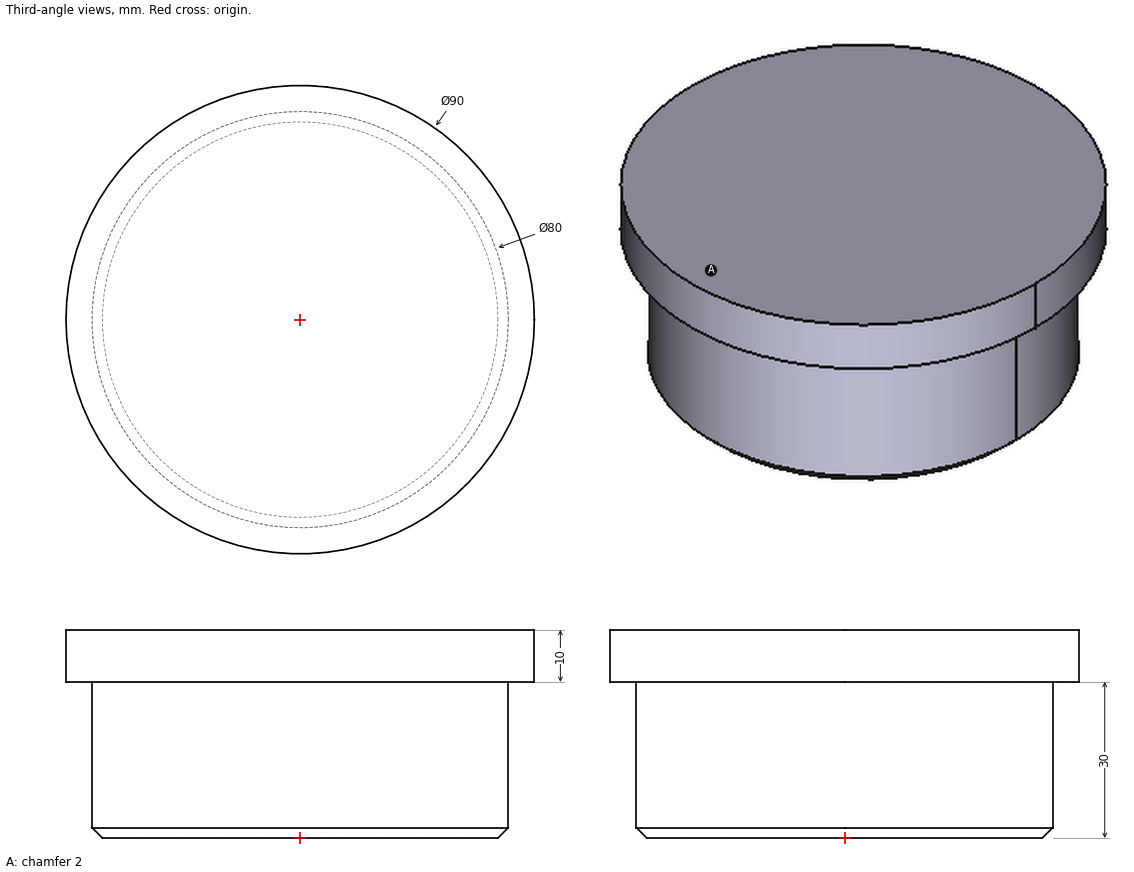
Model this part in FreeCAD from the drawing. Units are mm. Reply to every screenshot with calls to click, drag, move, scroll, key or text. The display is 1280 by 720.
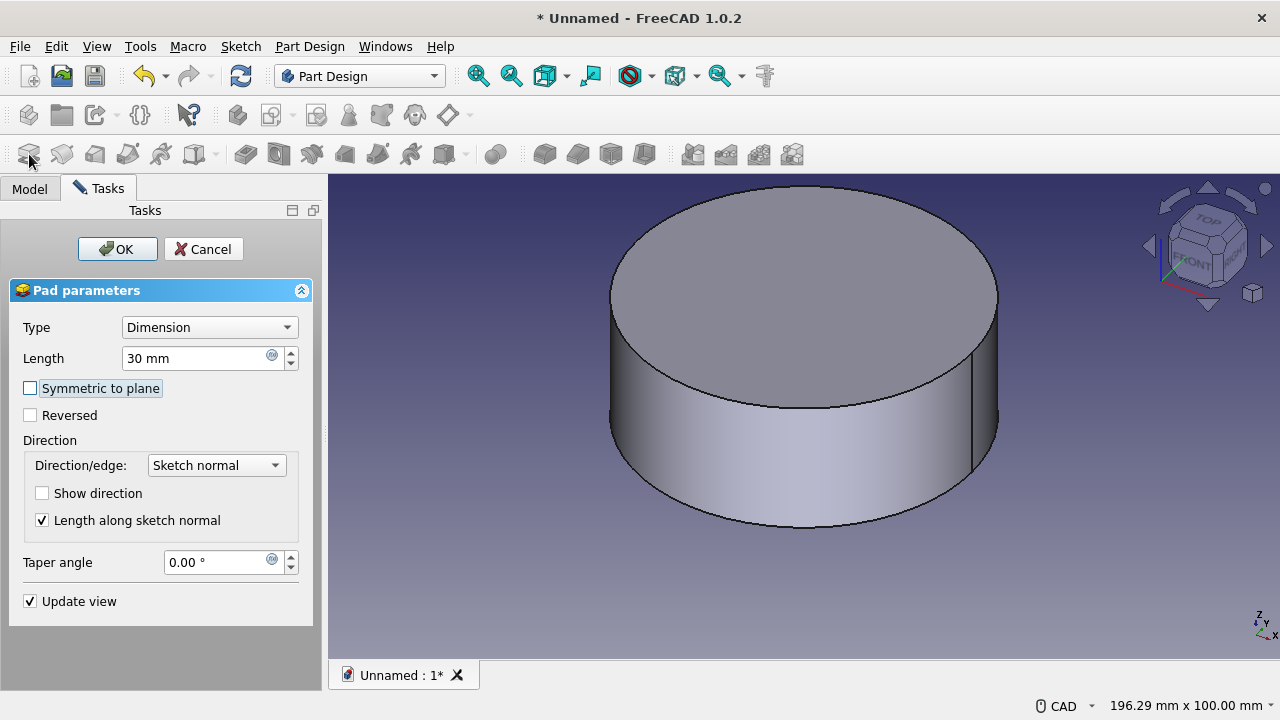
click(118, 249)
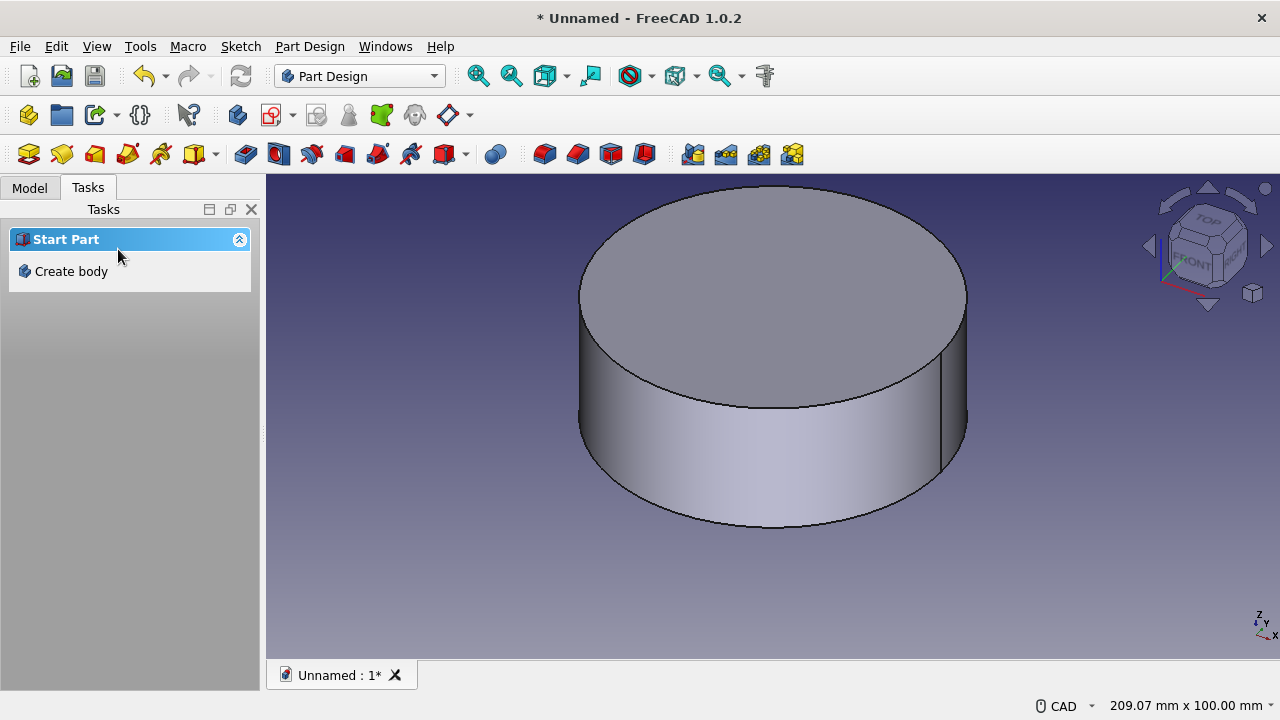
click(479, 76)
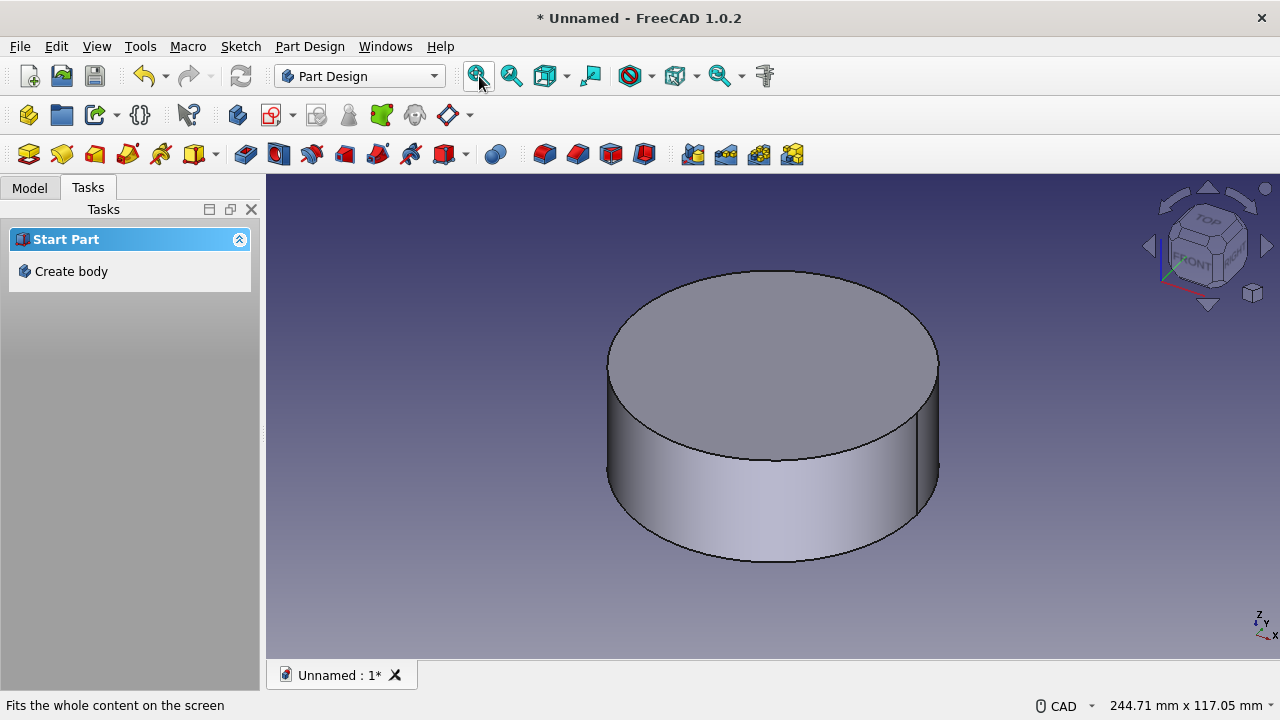
click(773, 365)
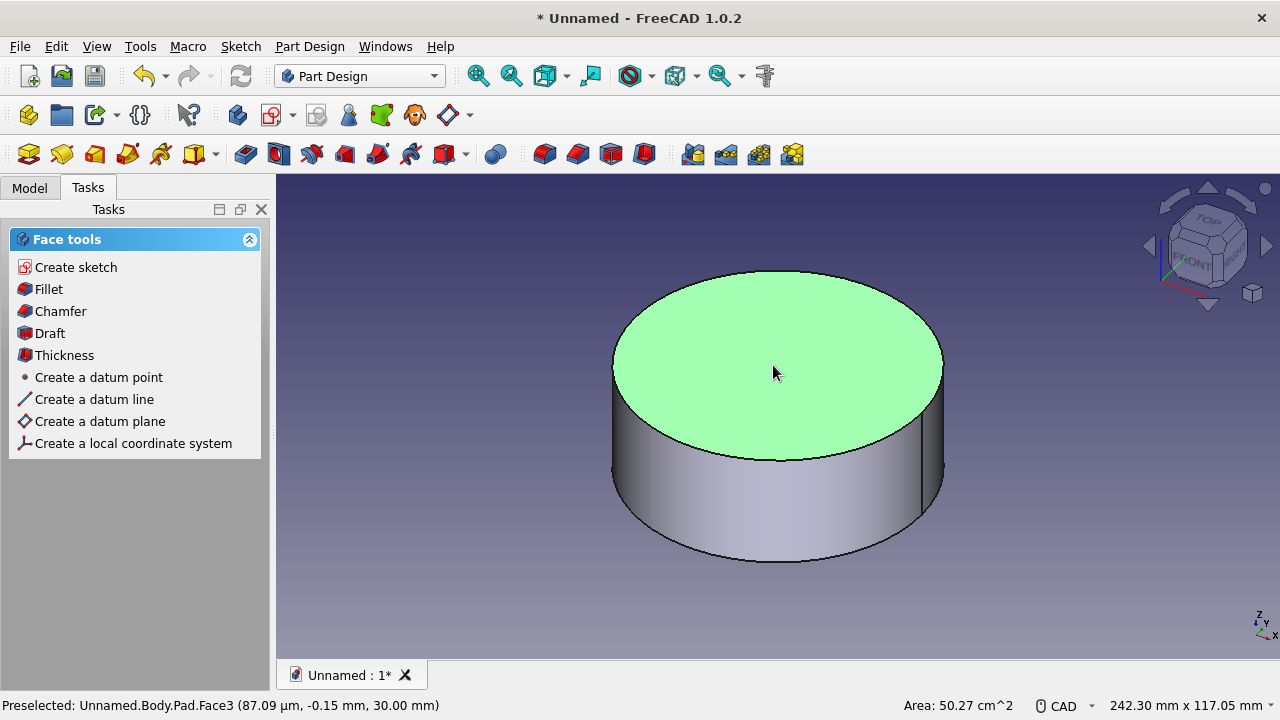
click(270, 116)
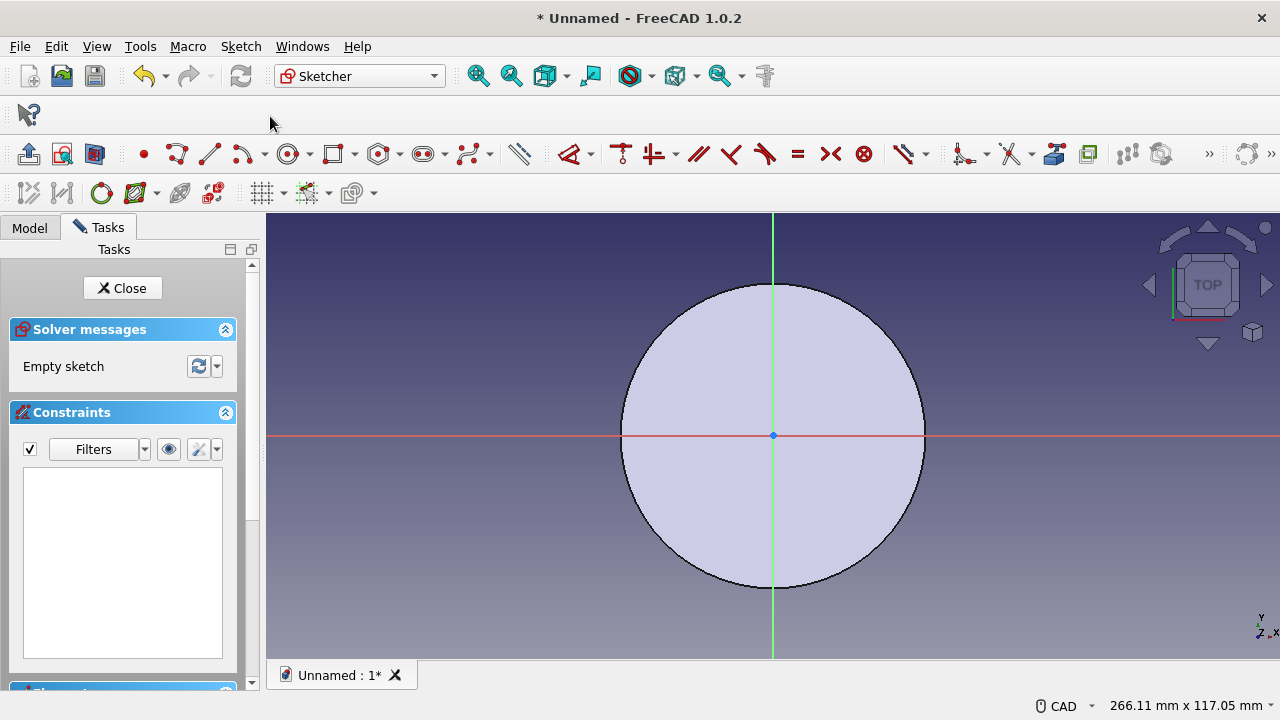
scroll(395, 436, down, 1)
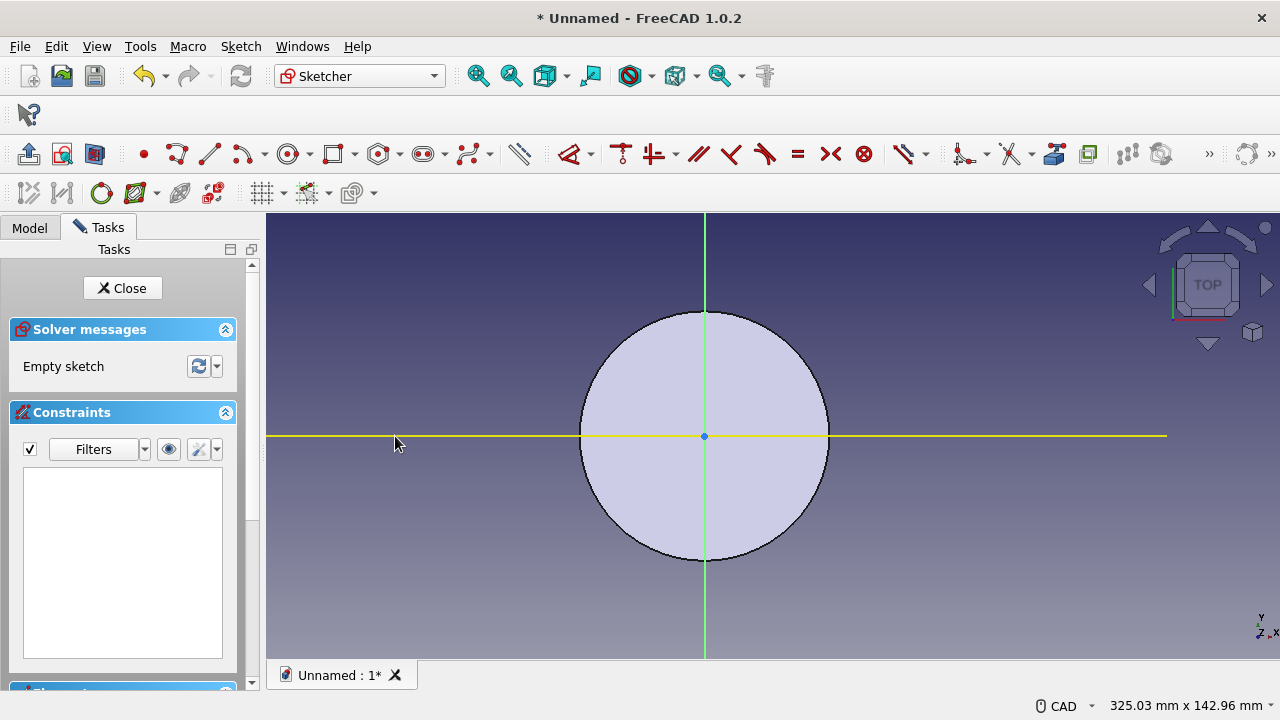
click(288, 154)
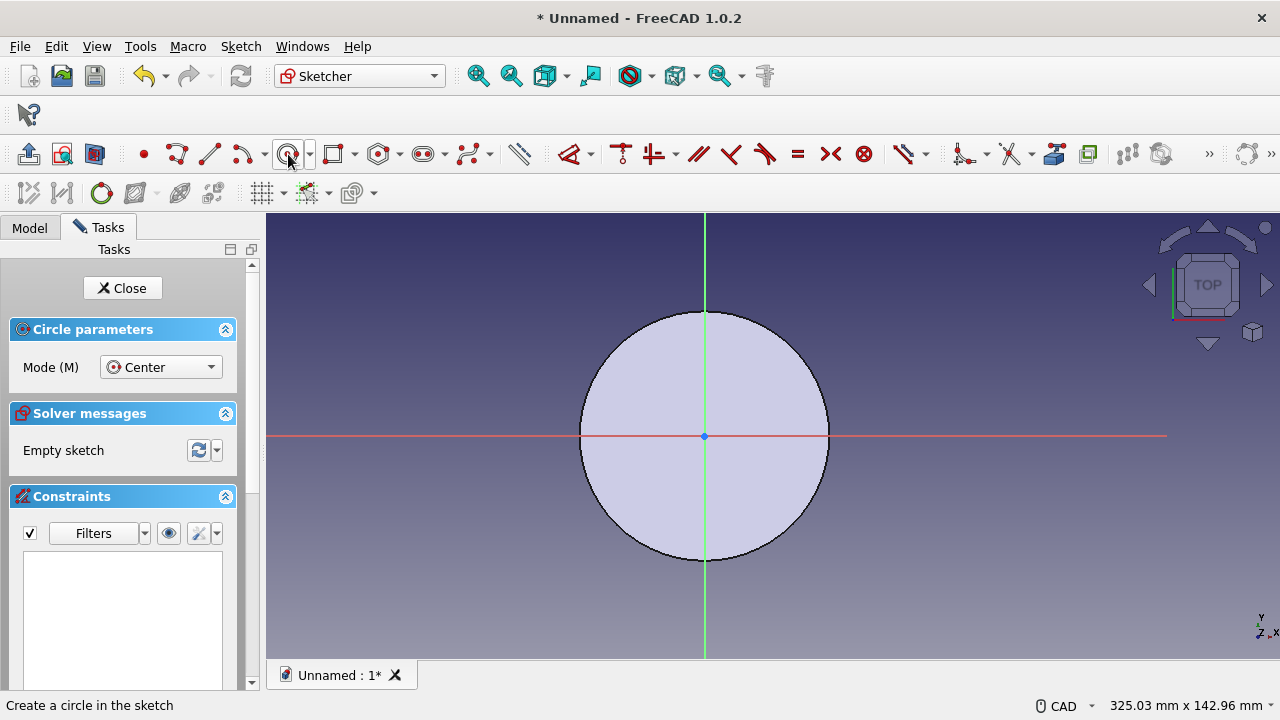
click(705, 436)
move(804, 337)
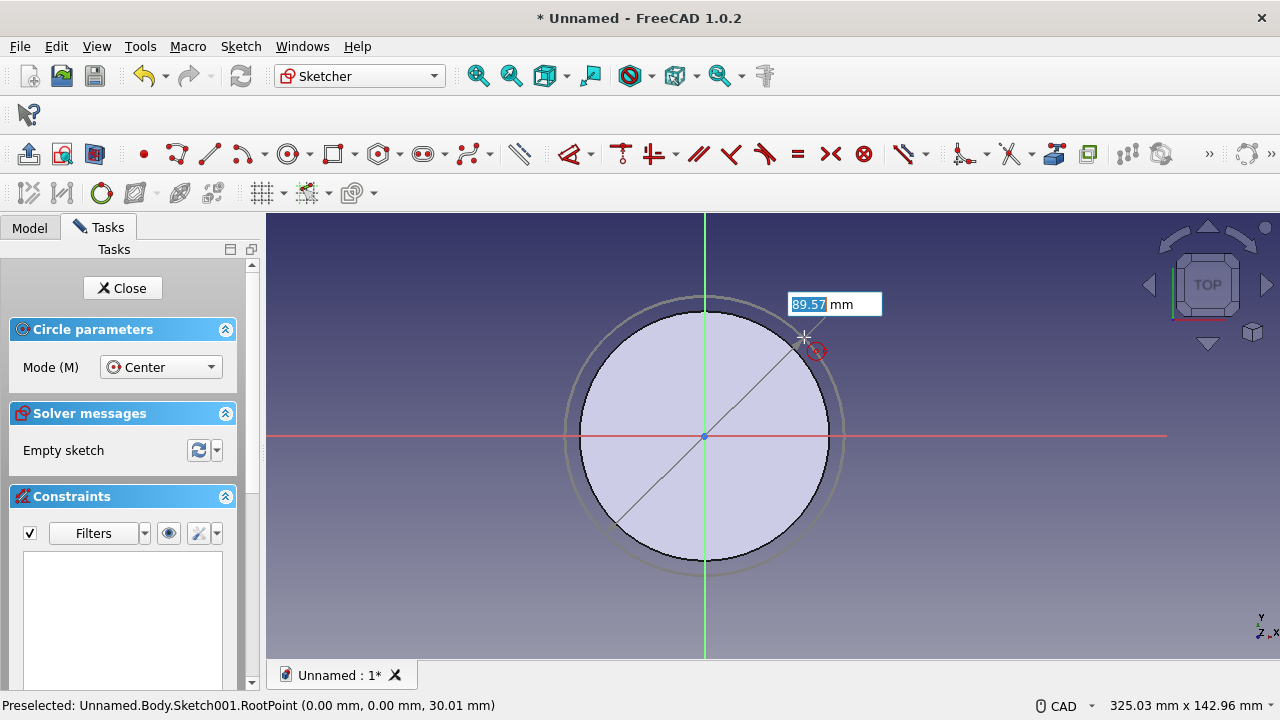
text(90)
key(Return)
key(Escape)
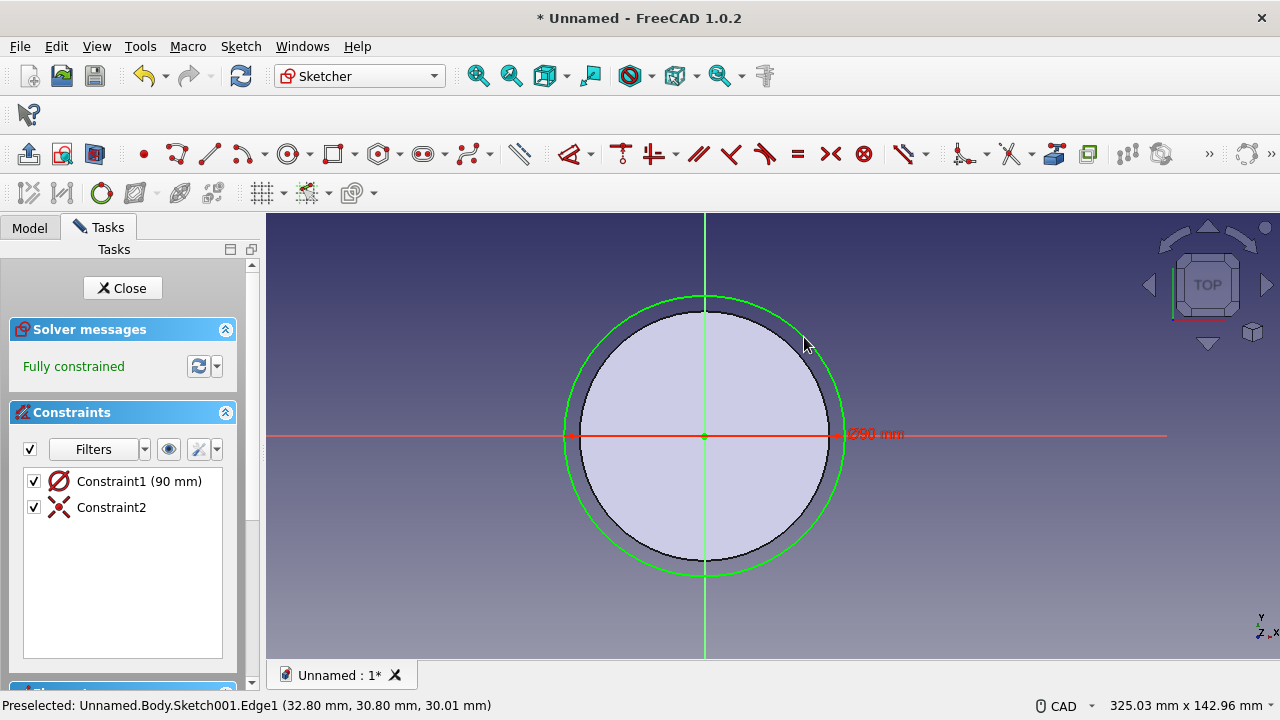
click(123, 288)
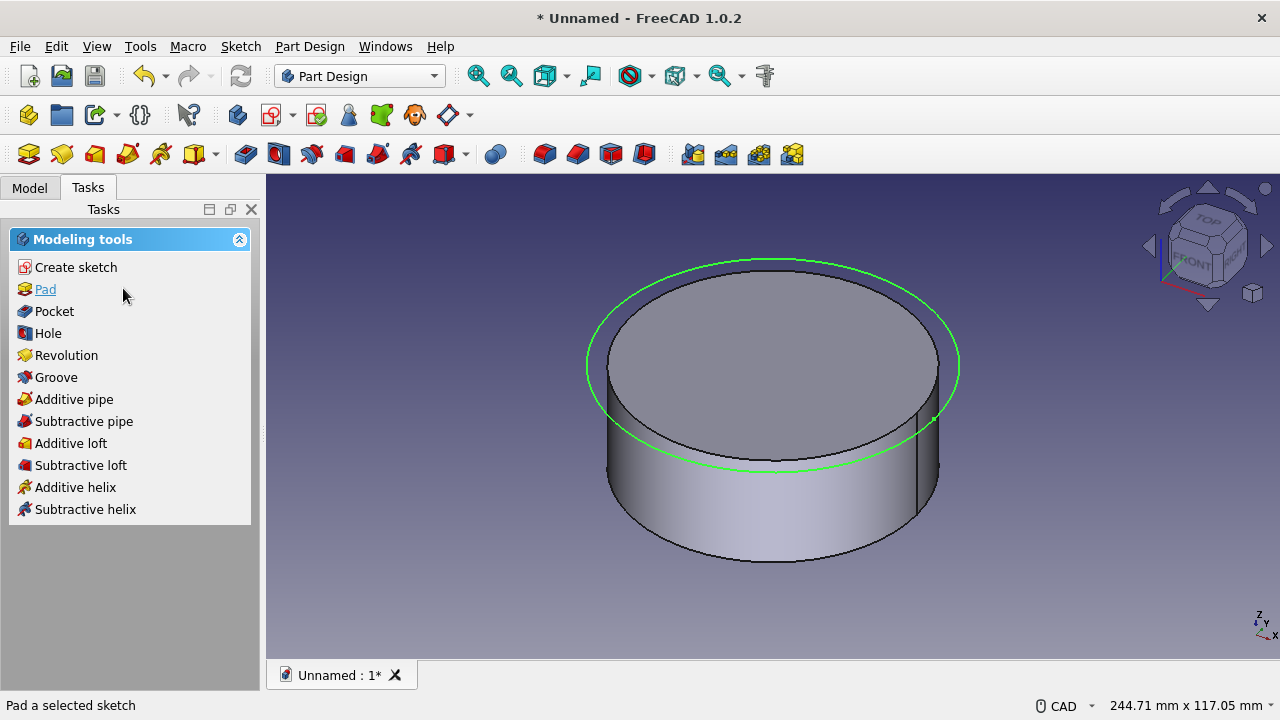
click(29, 154)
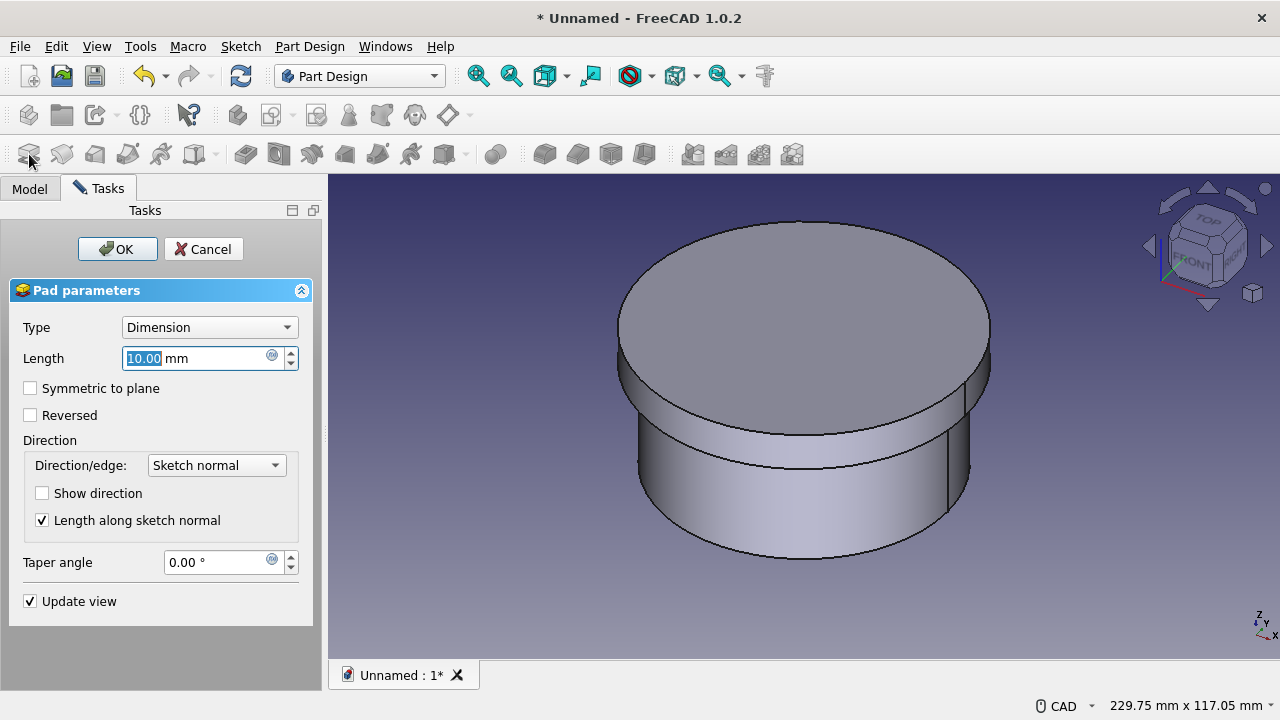
text(10)
key(Tab)